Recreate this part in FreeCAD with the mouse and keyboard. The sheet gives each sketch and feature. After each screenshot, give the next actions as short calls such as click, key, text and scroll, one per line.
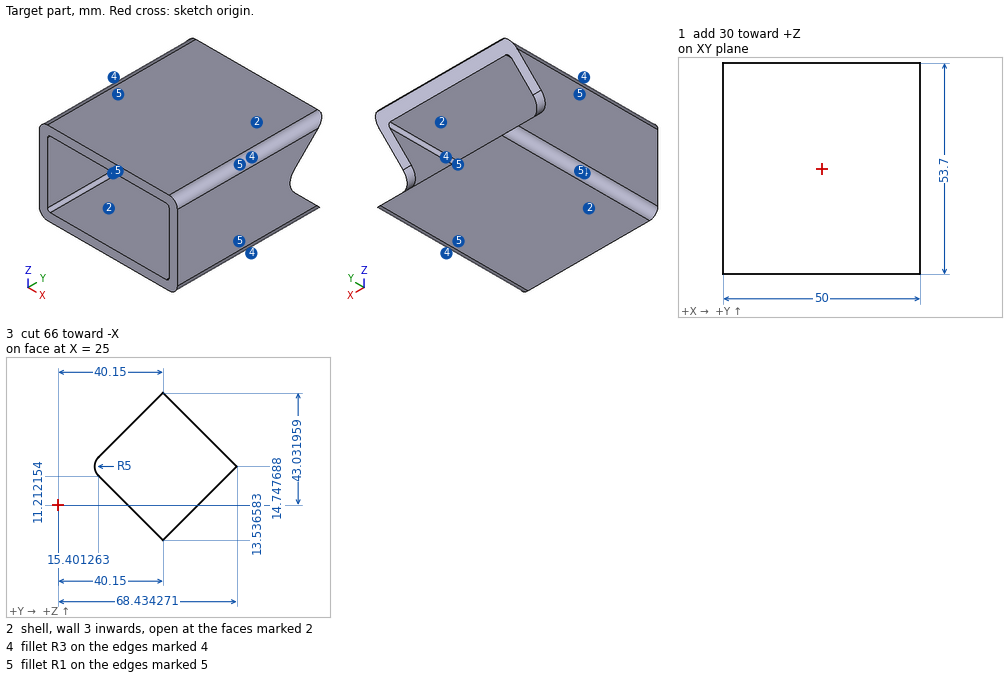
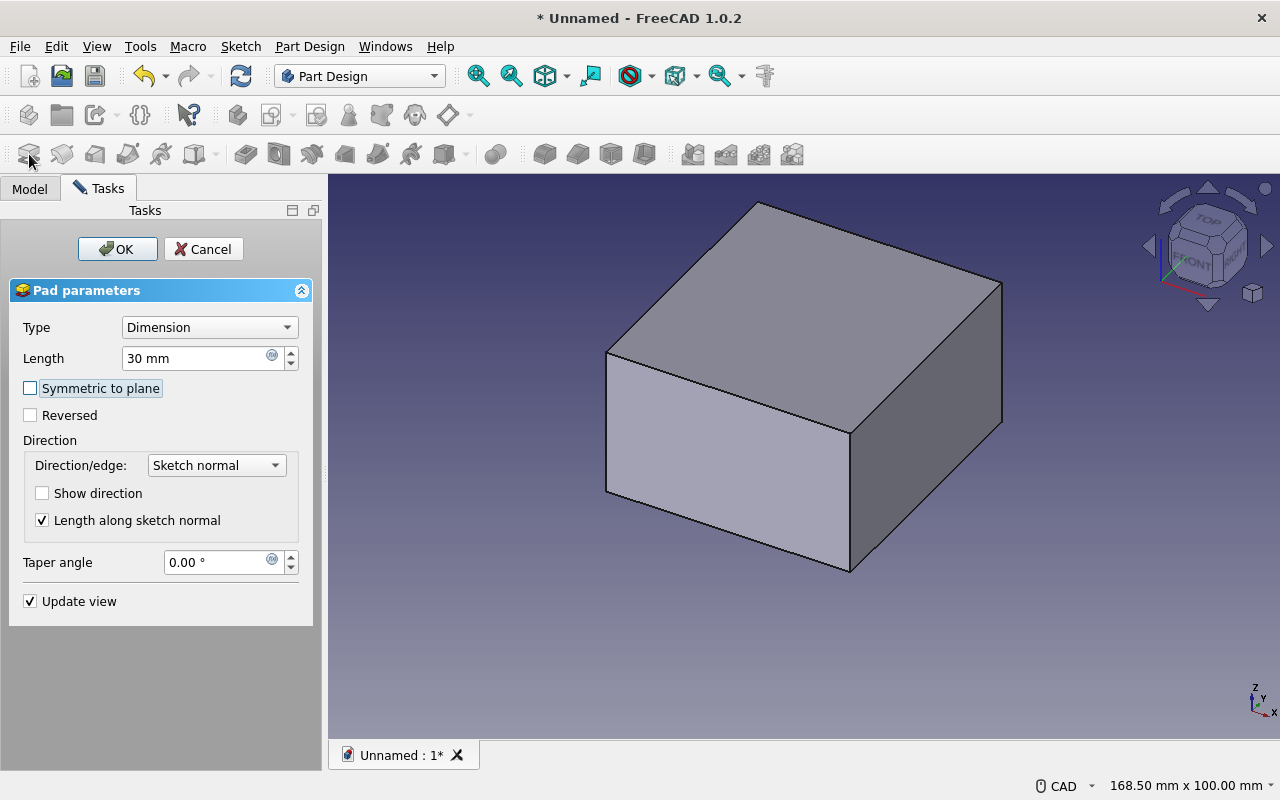
click(118, 249)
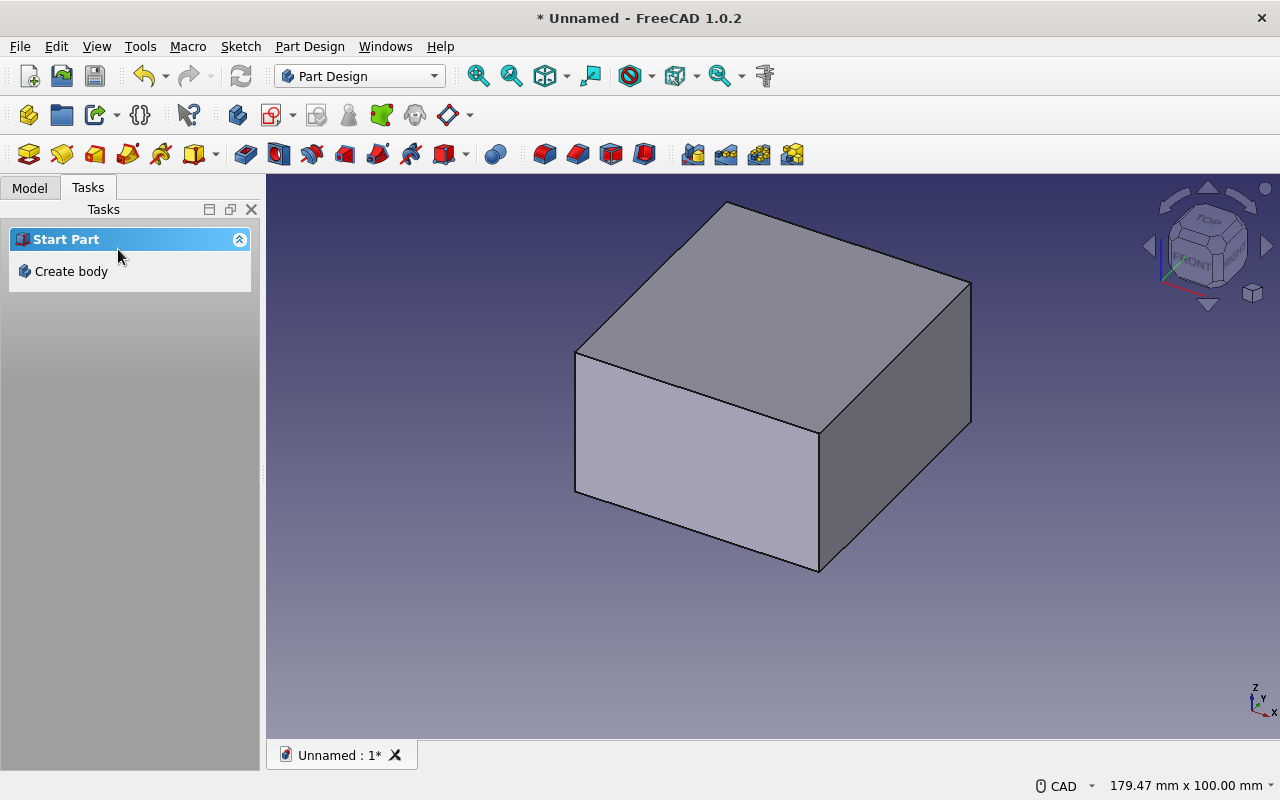
click(732, 473)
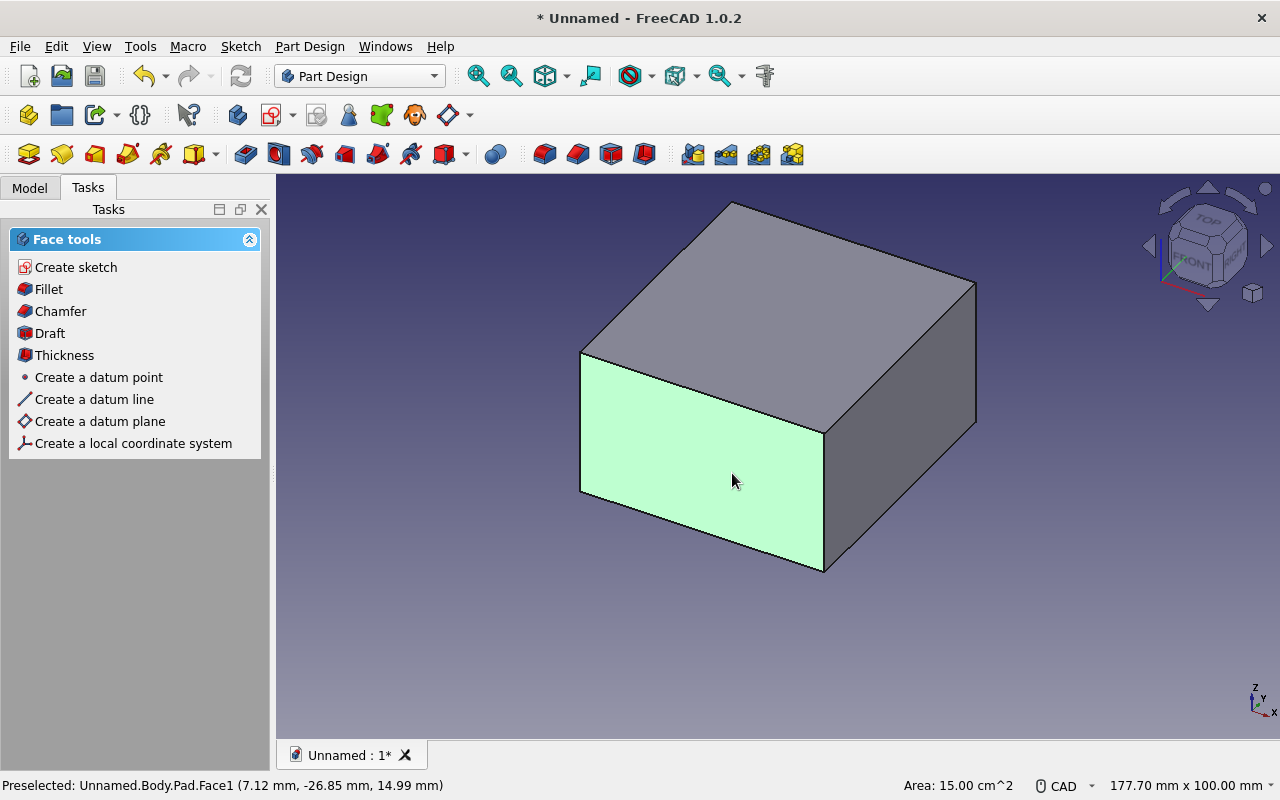
key(0)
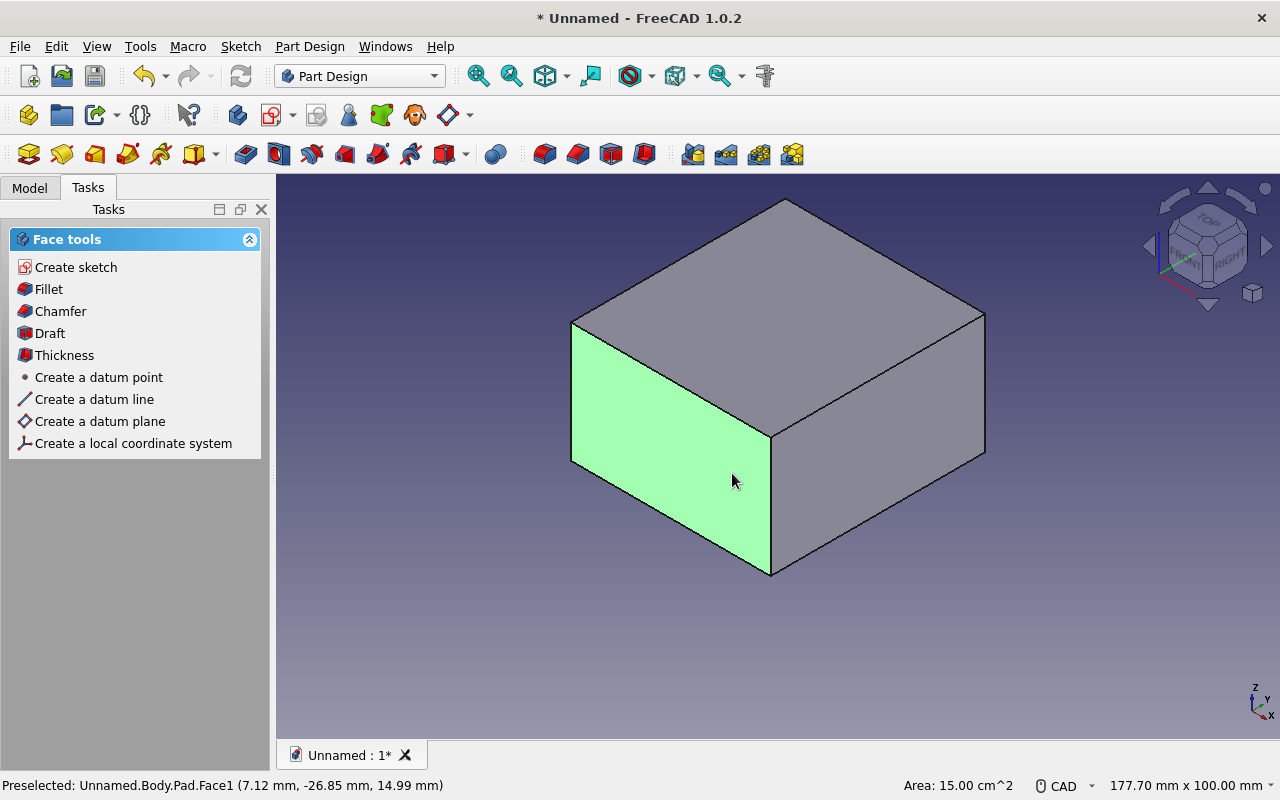
key(2)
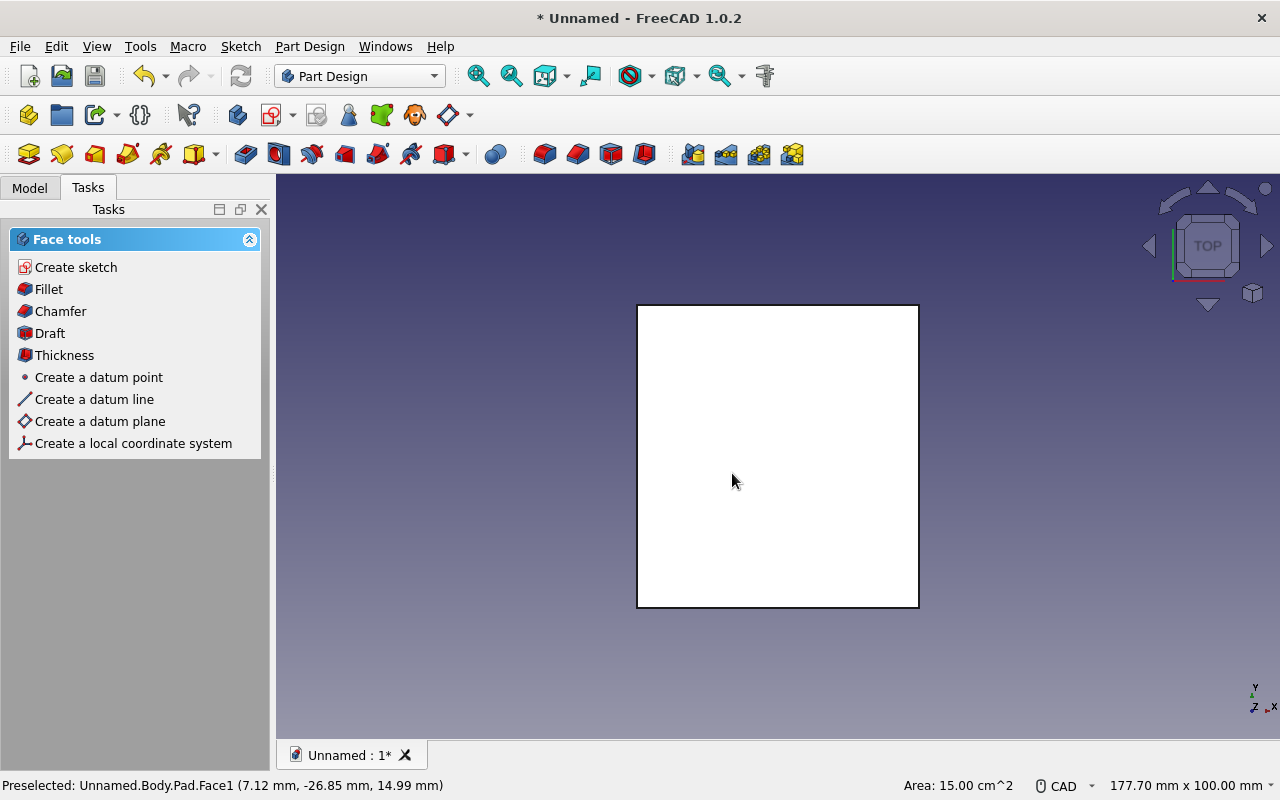
key(1)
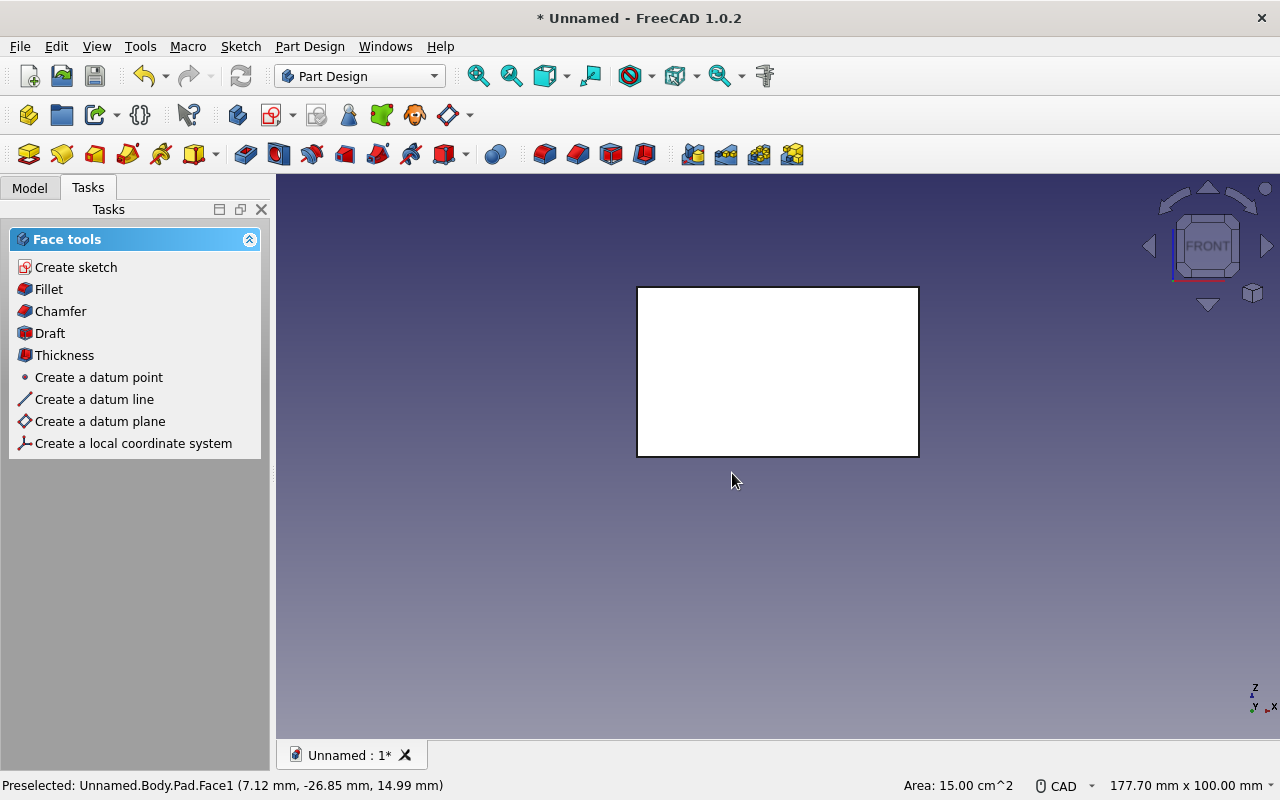
click(479, 76)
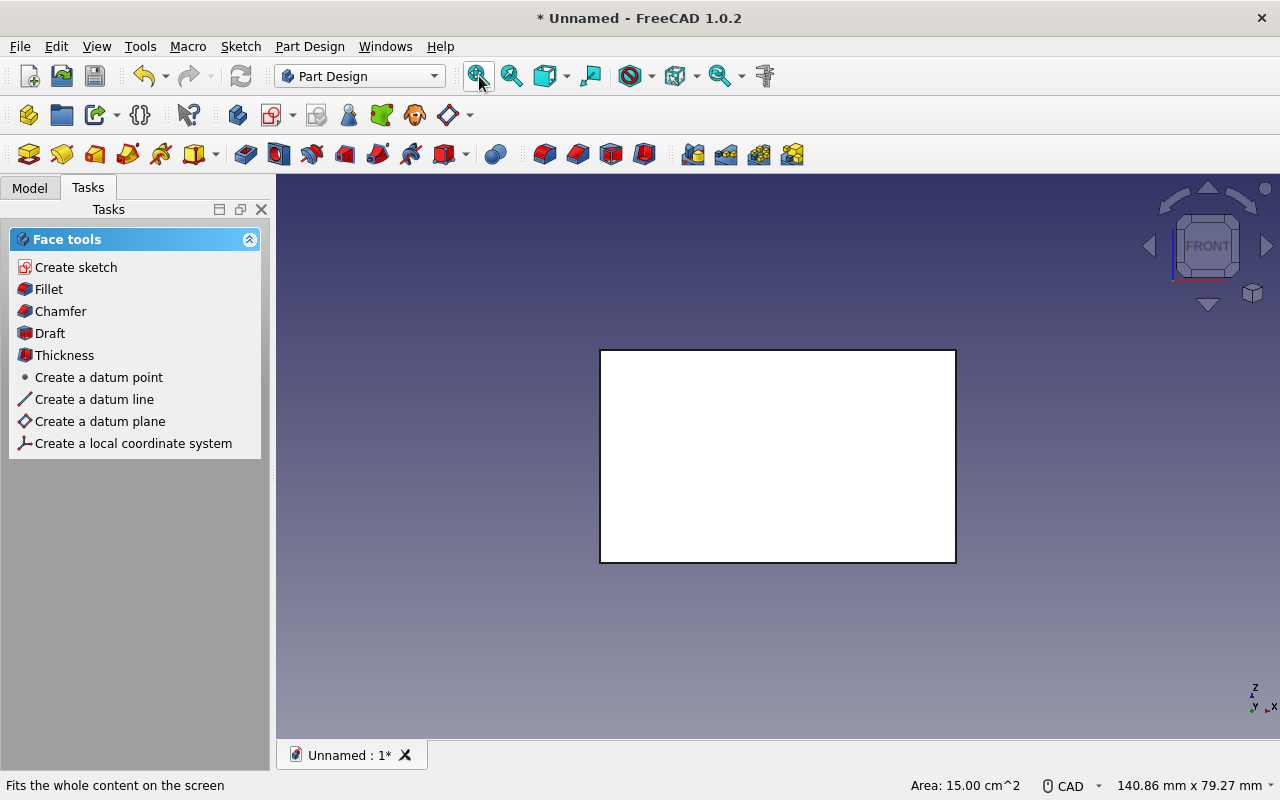
key(3)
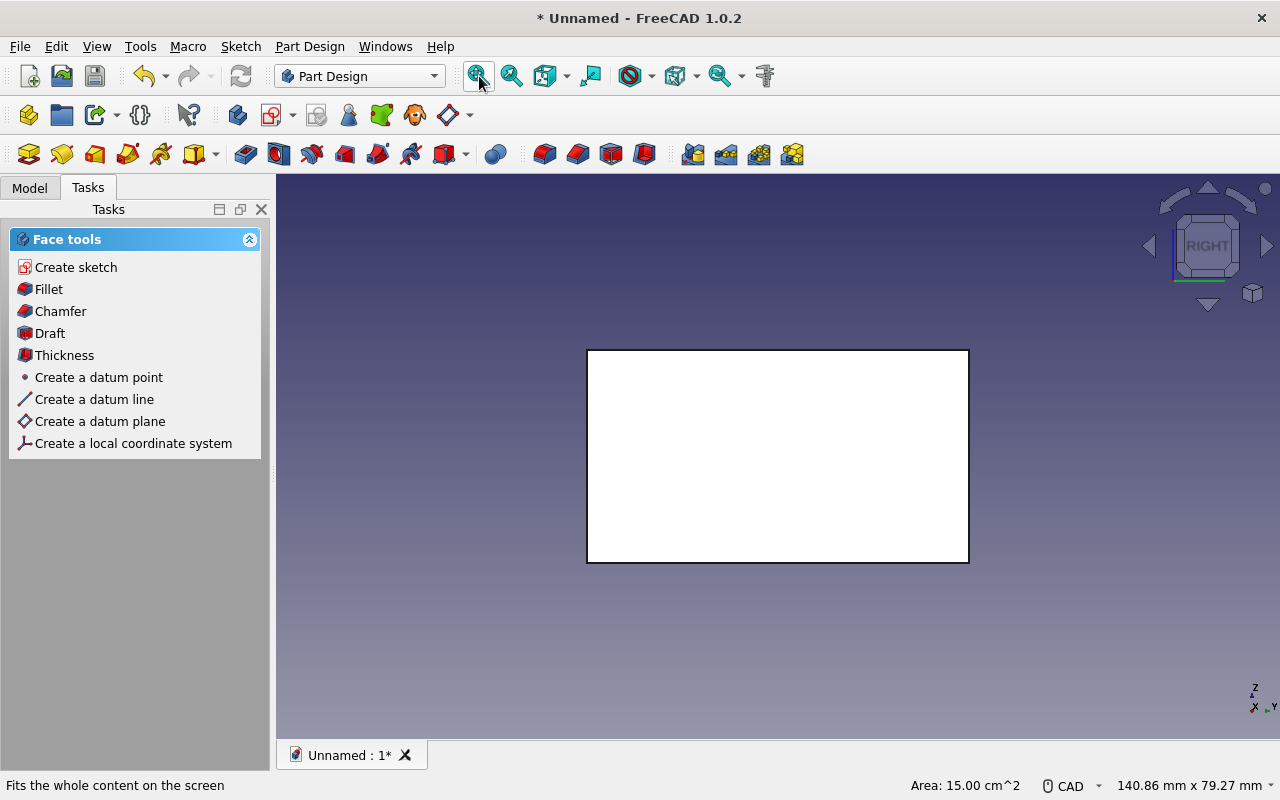
key(v)
key(f)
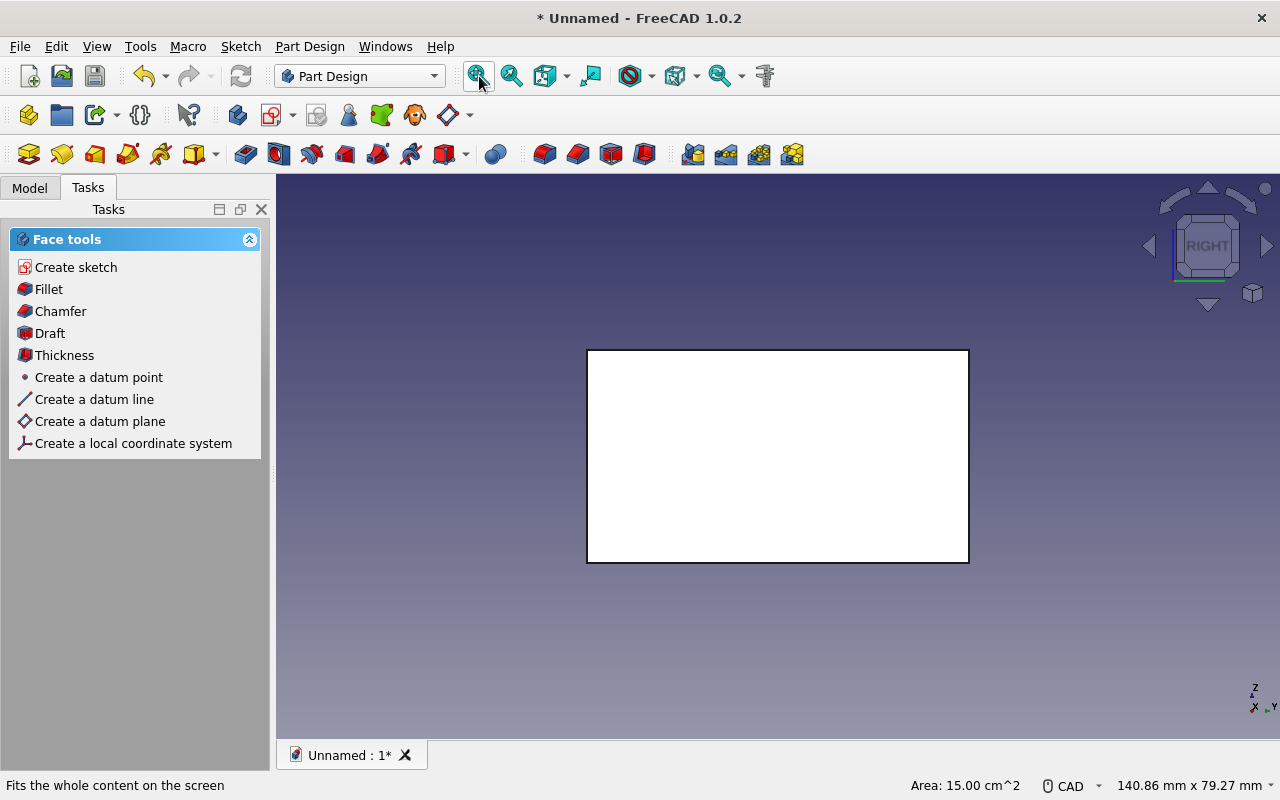
key(5)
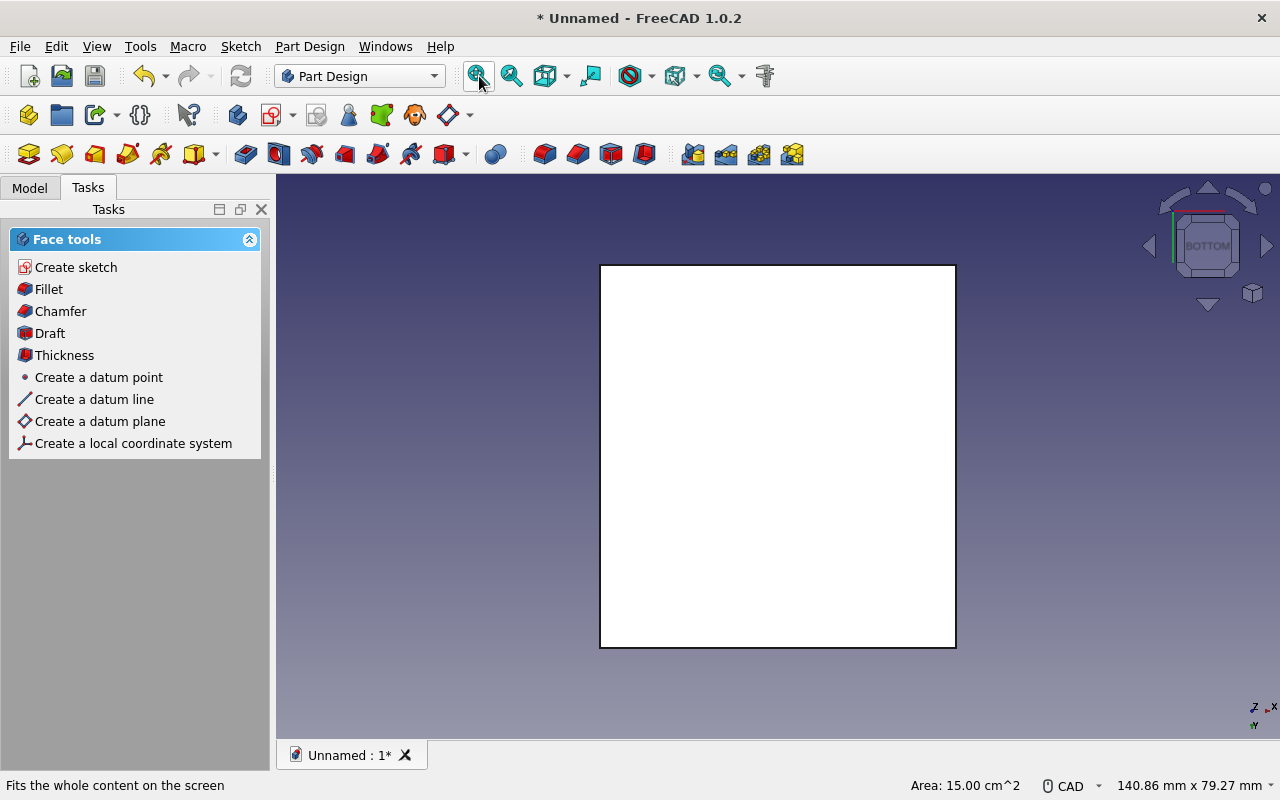
key(4)